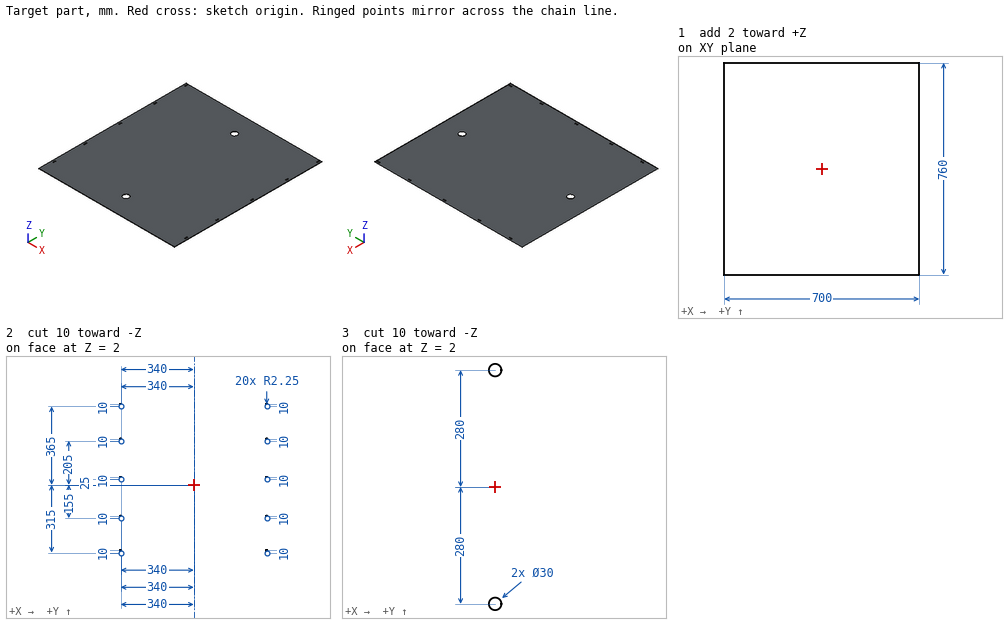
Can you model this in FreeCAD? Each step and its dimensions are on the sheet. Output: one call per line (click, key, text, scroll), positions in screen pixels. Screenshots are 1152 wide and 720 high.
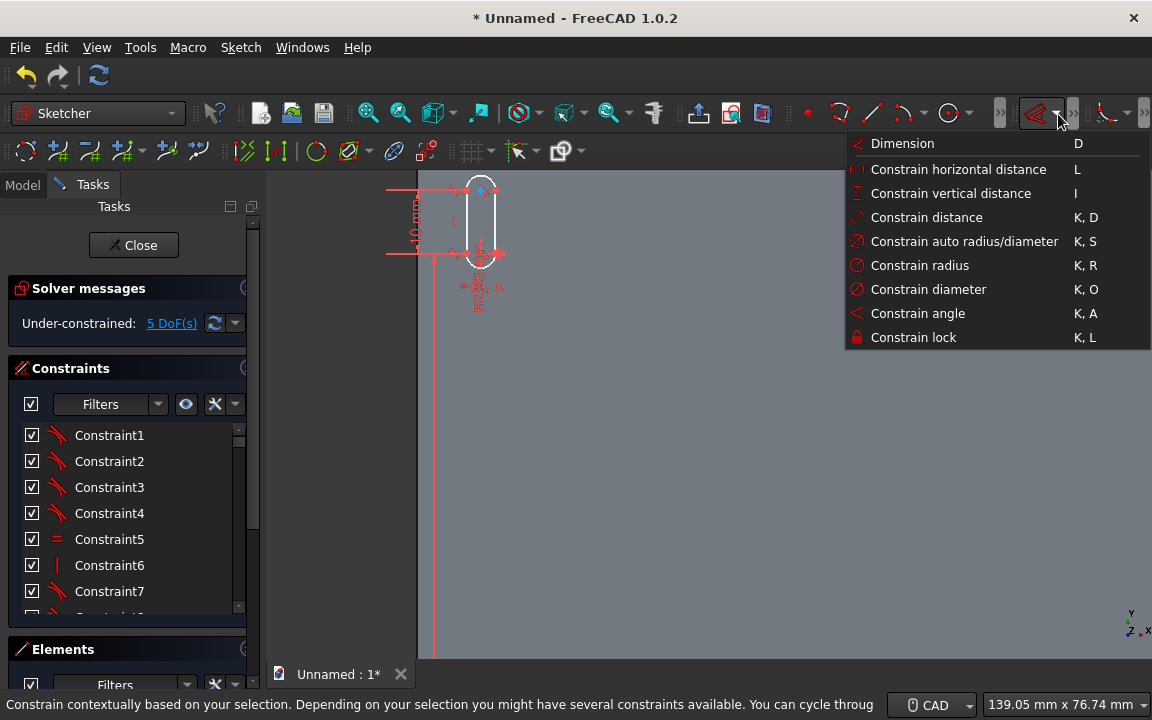
click(998, 169)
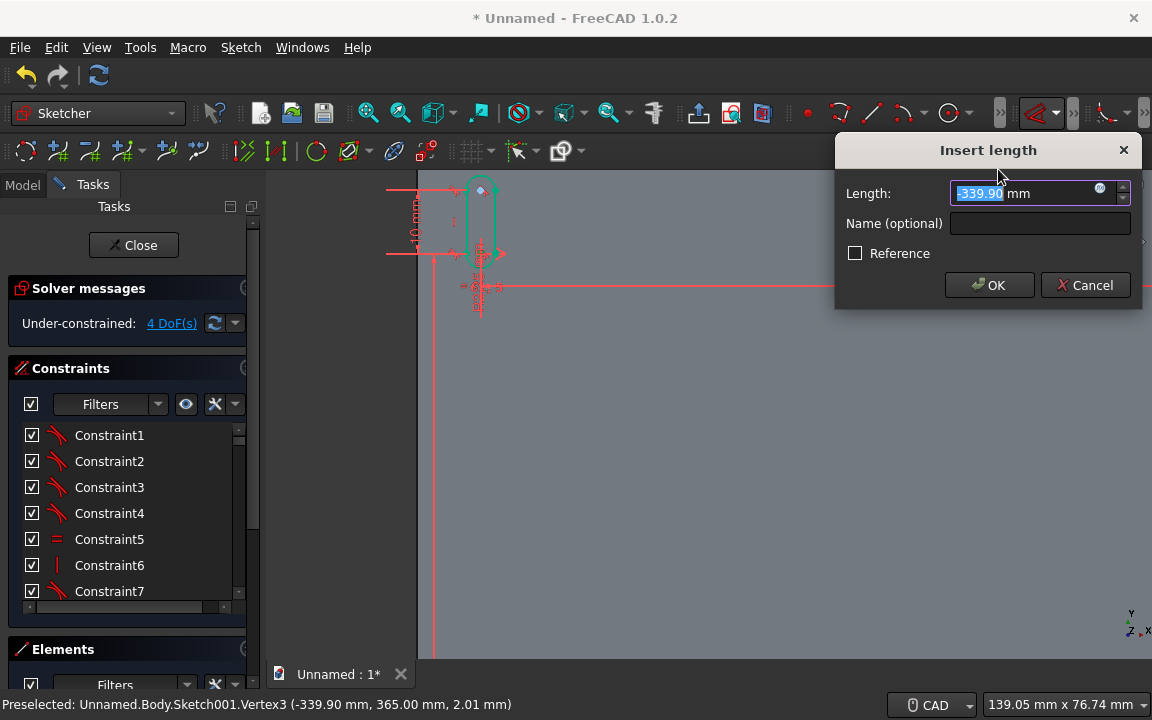
text(-340)
key(Return)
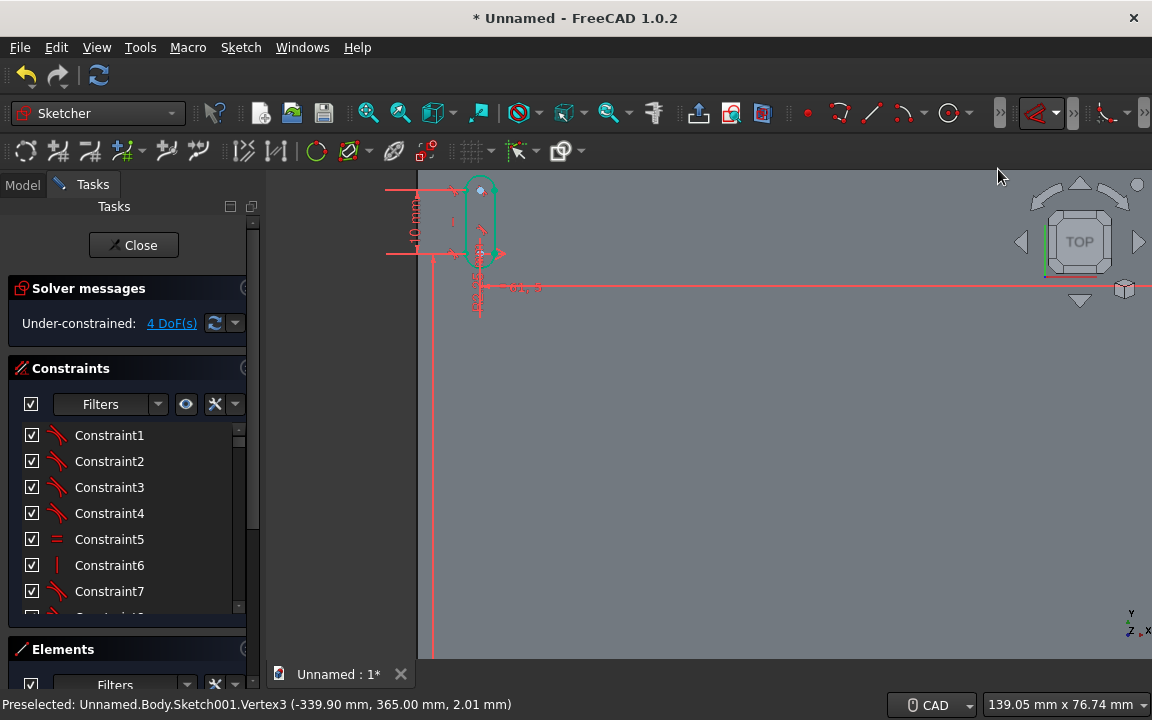
scroll(480, 256, down, 13)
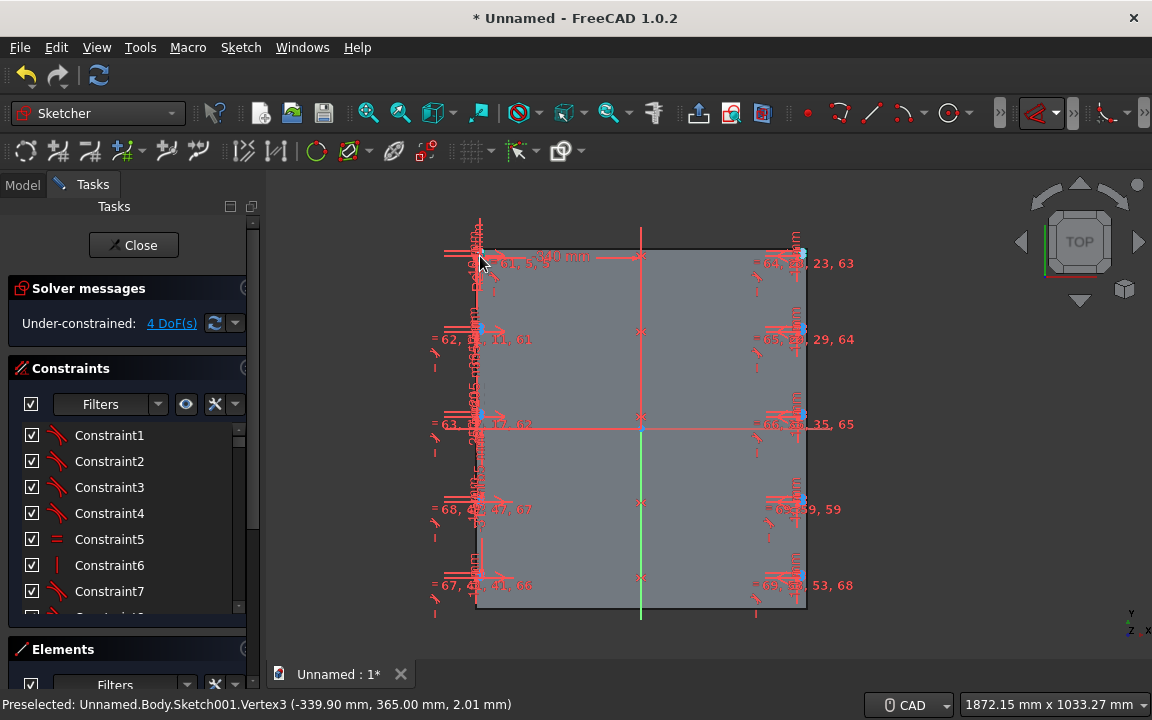
scroll(480, 332, up, 13)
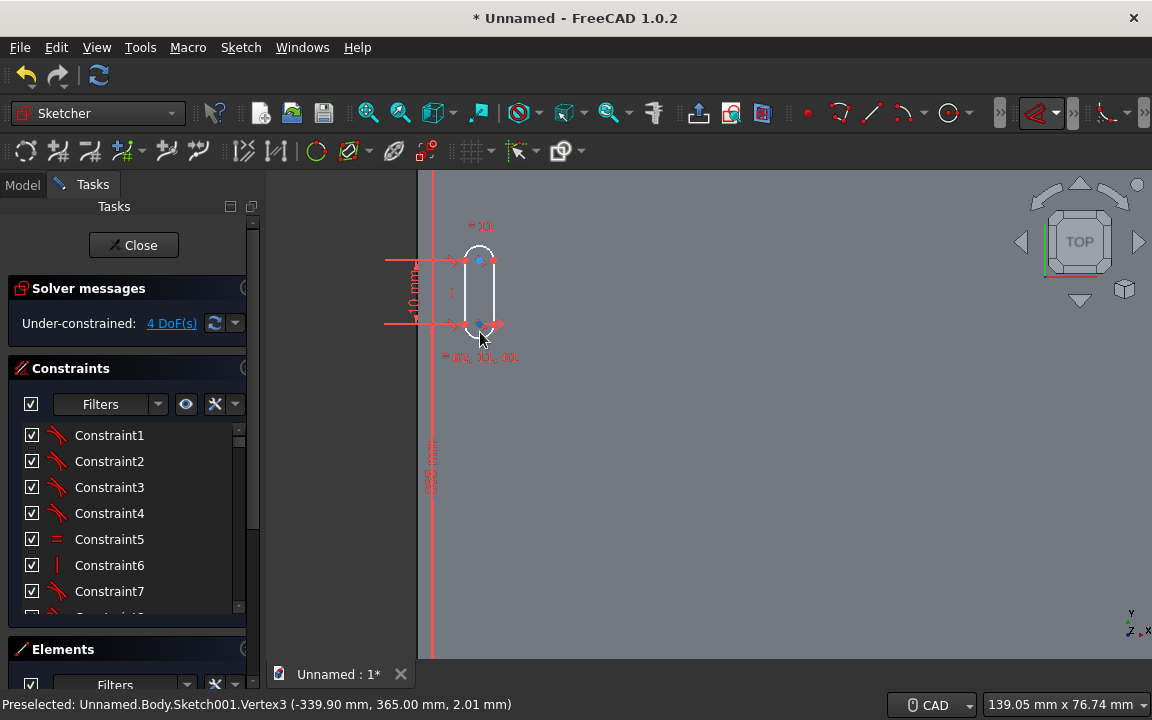
click(479, 324)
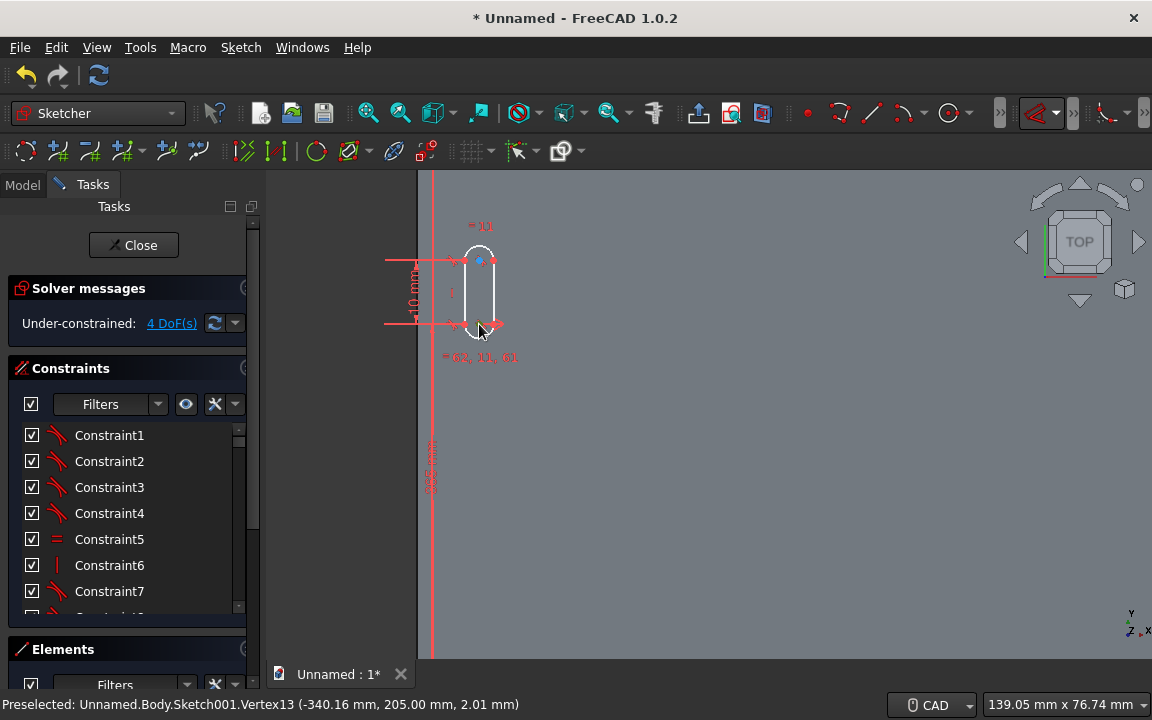
click(1058, 114)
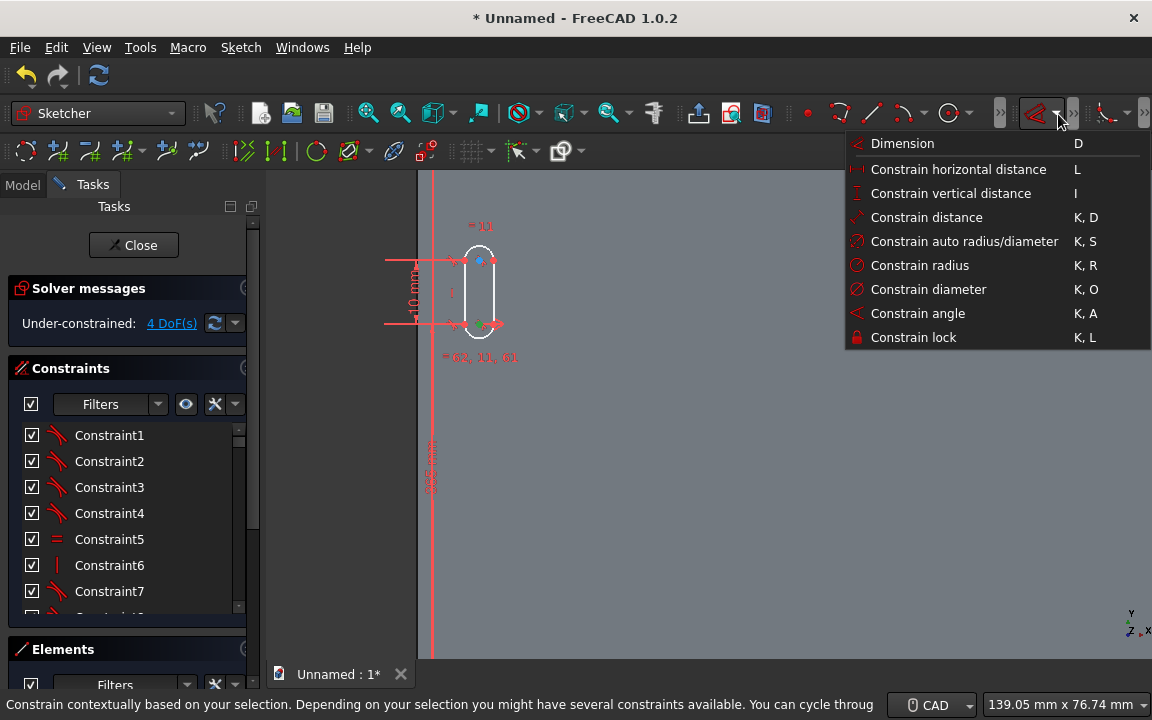
click(998, 169)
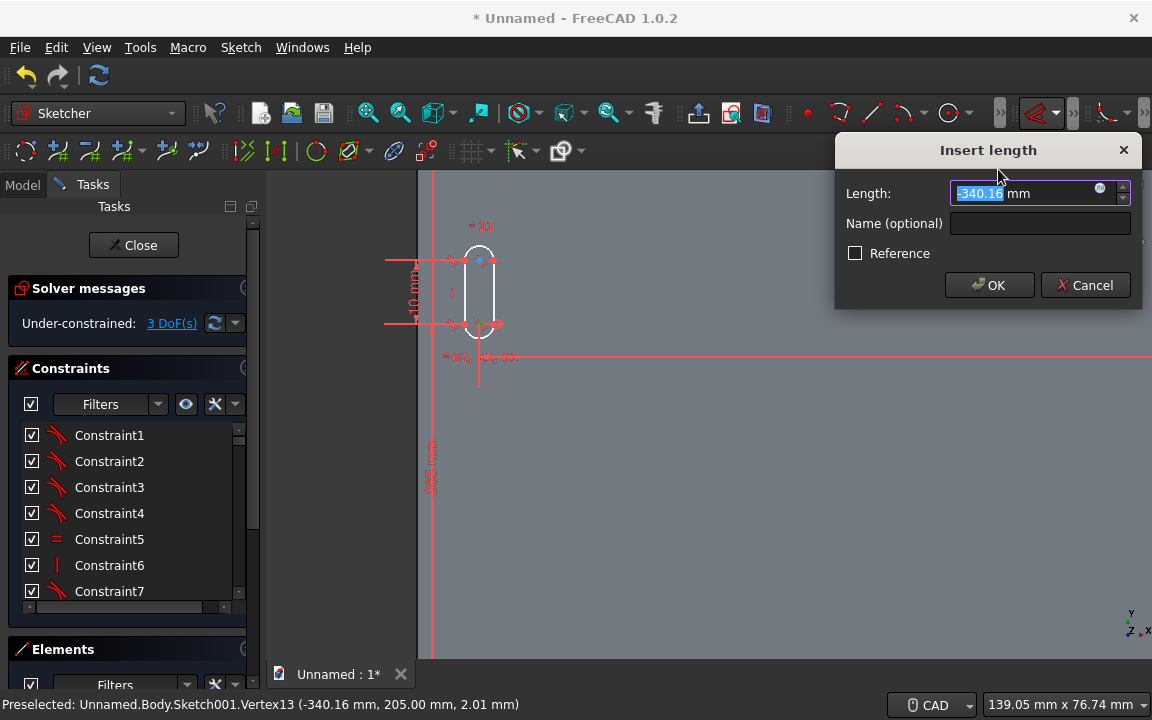
text(-340)
key(Return)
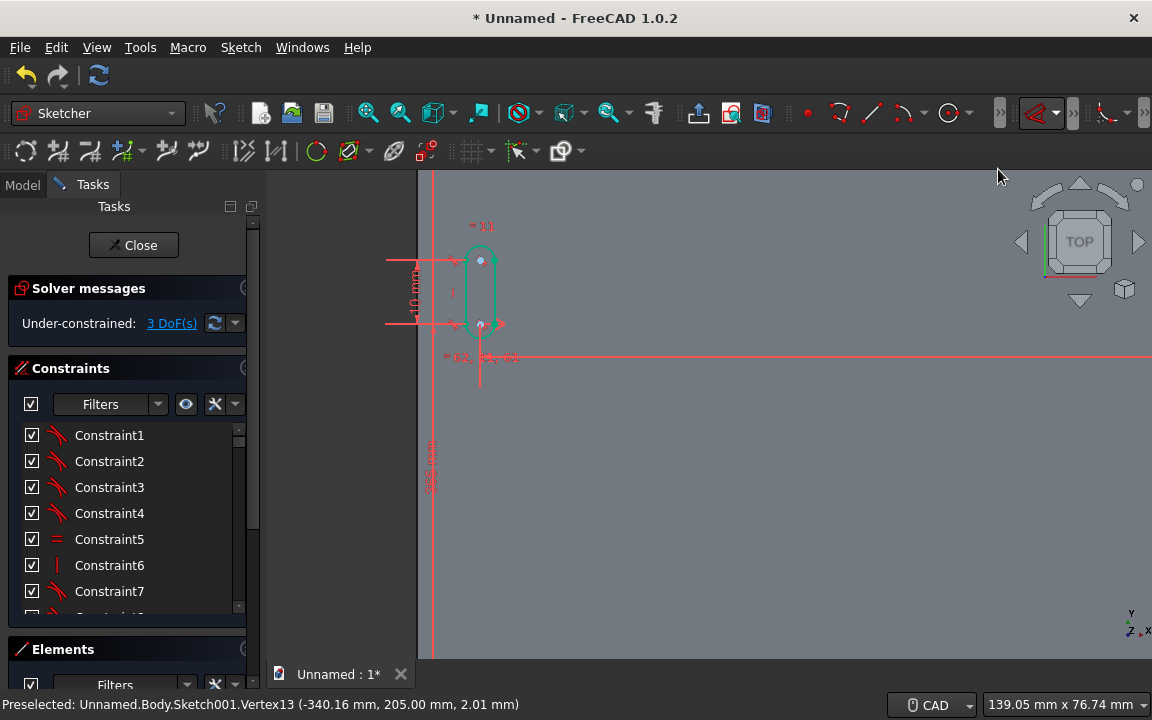
scroll(480, 332, down, 13)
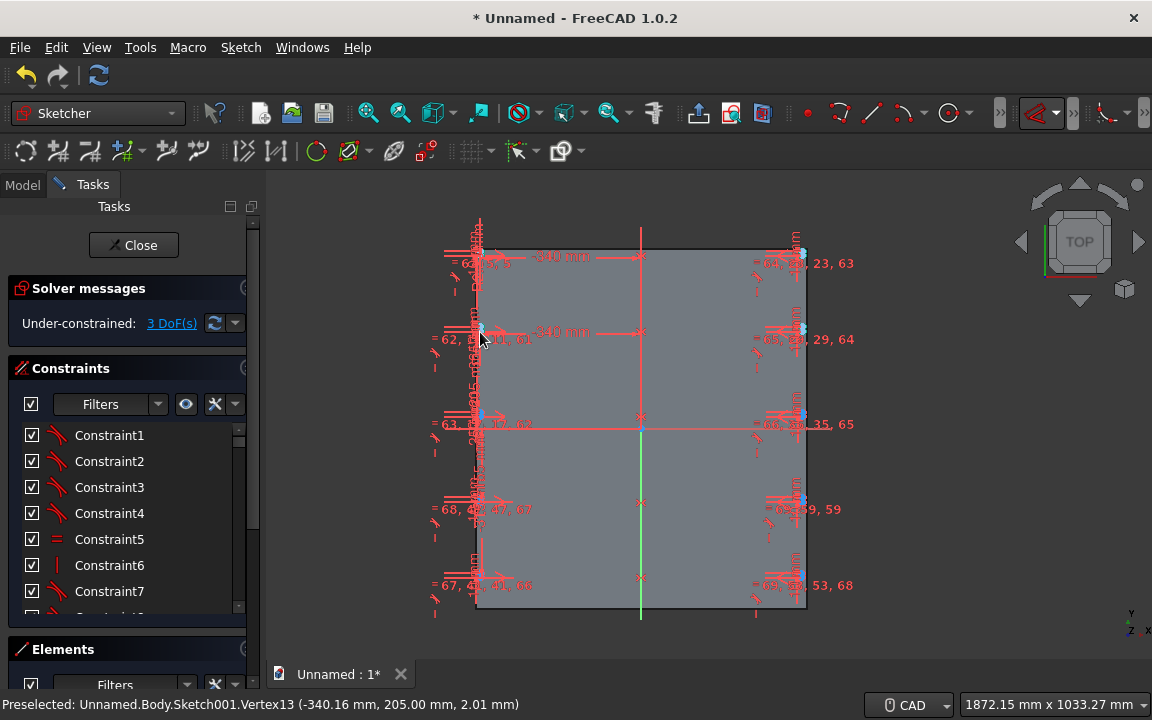
scroll(480, 417, up, 13)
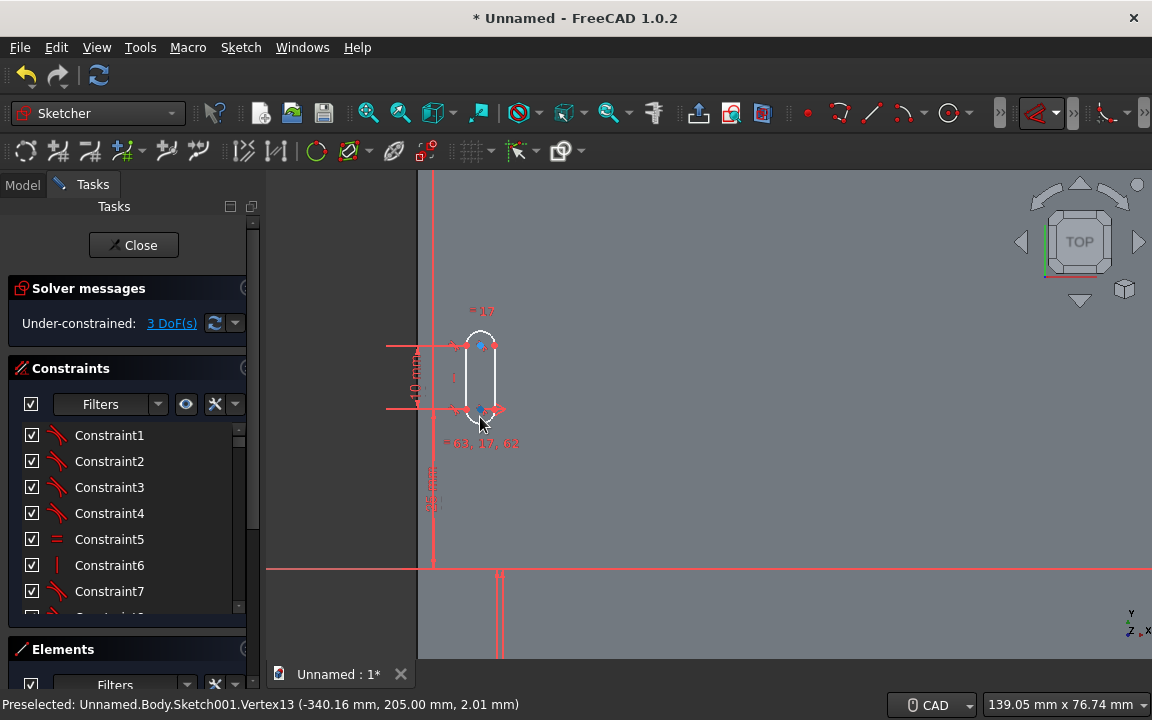
click(481, 409)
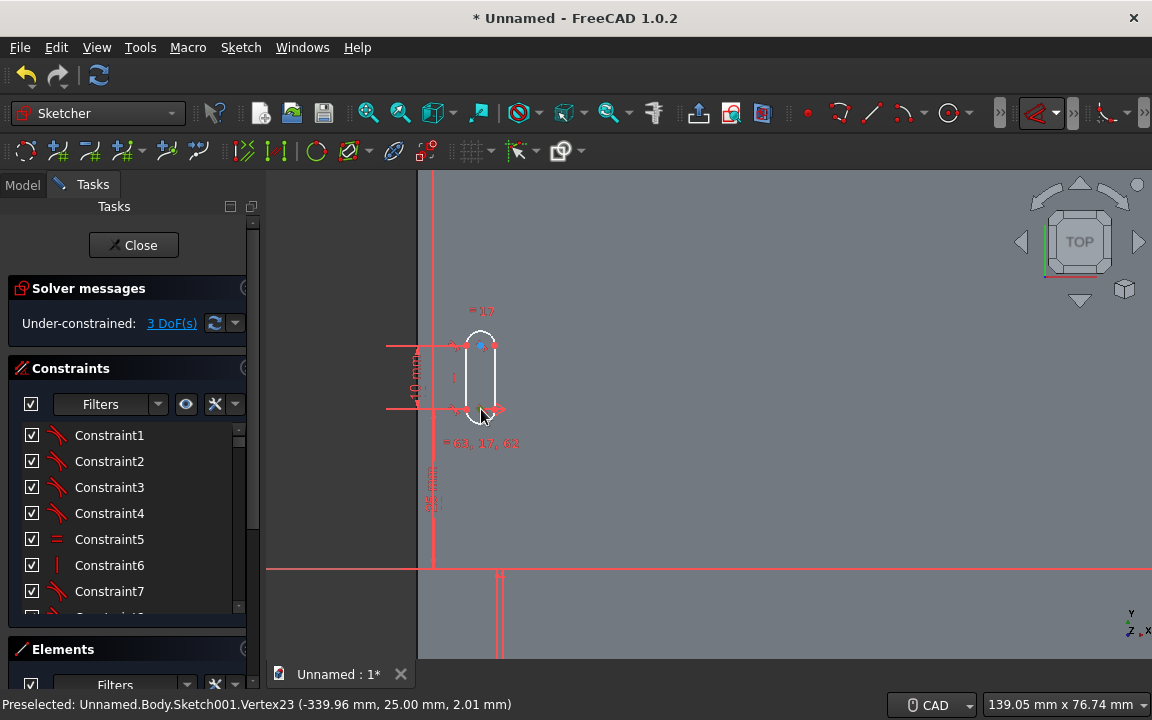
click(1058, 114)